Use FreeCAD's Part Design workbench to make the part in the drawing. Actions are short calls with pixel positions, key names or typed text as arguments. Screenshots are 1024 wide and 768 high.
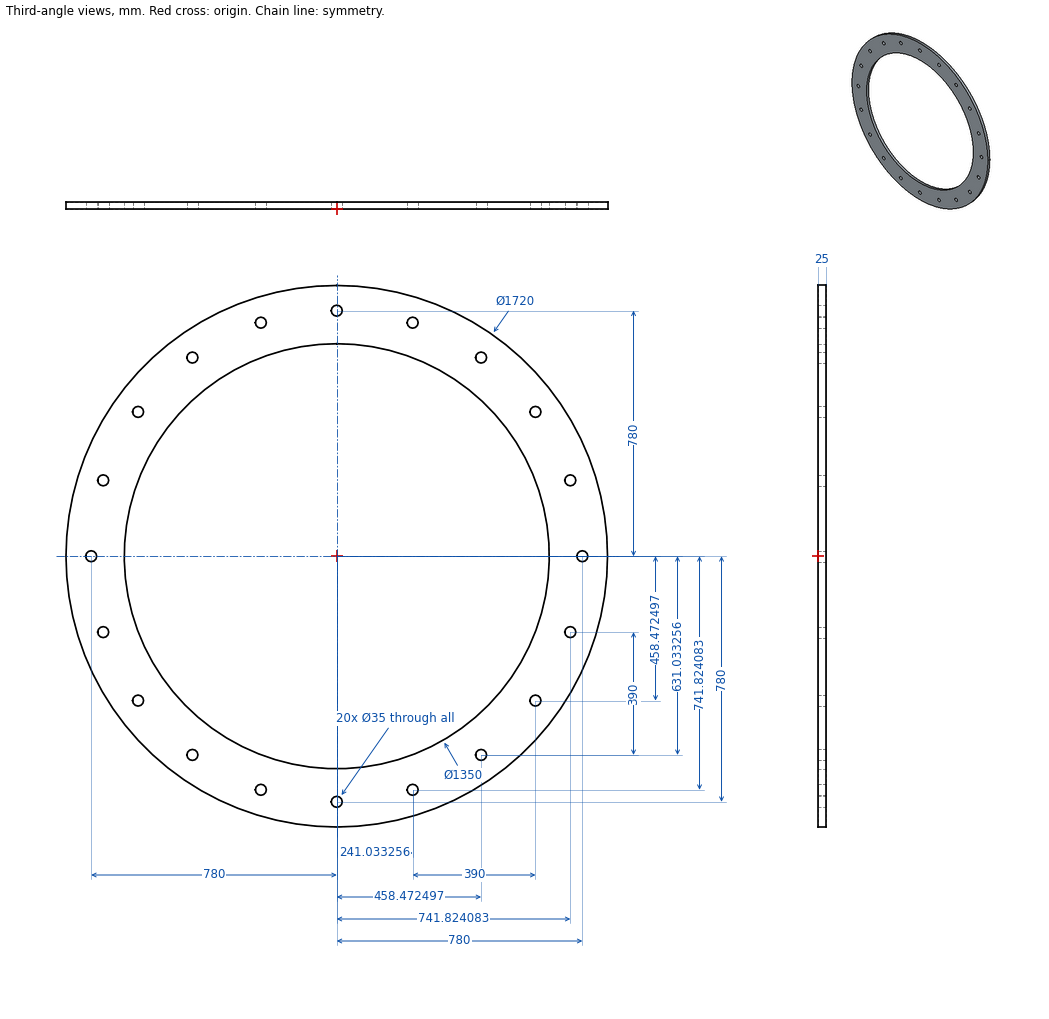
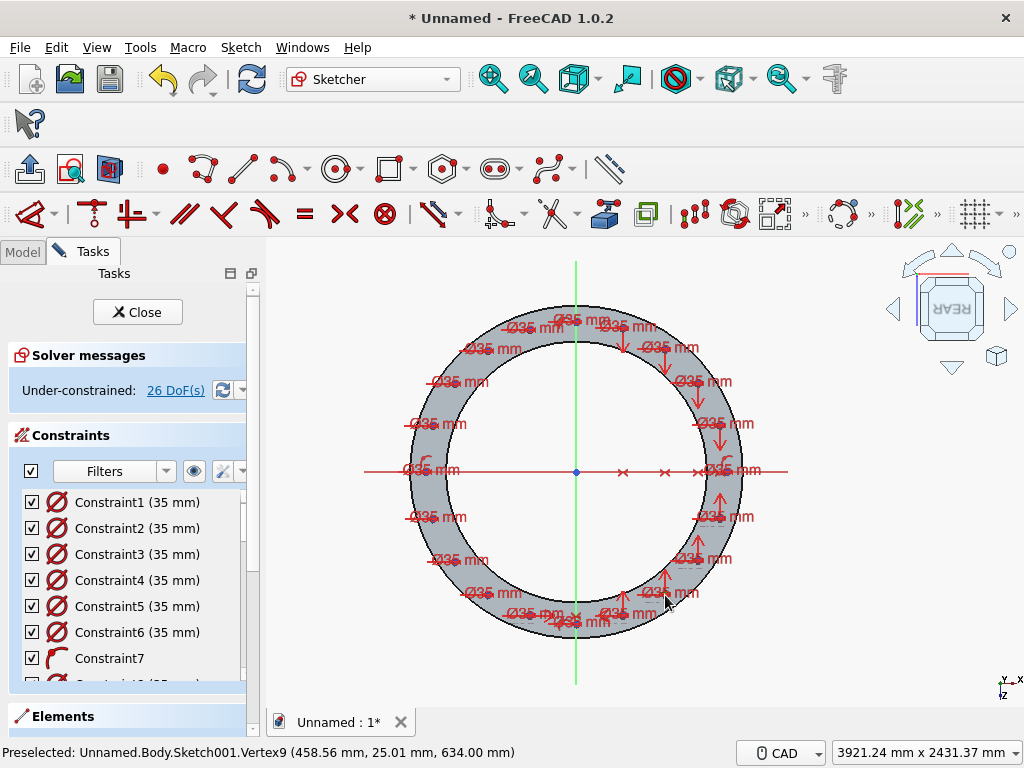
click(488, 595)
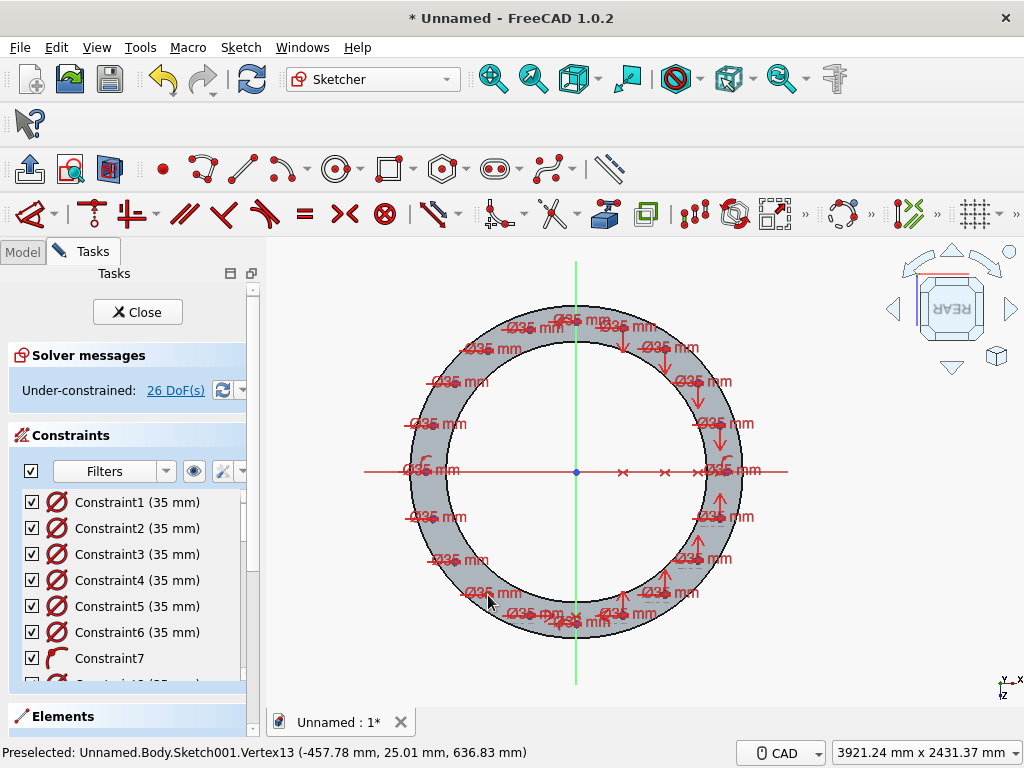
click(576, 590)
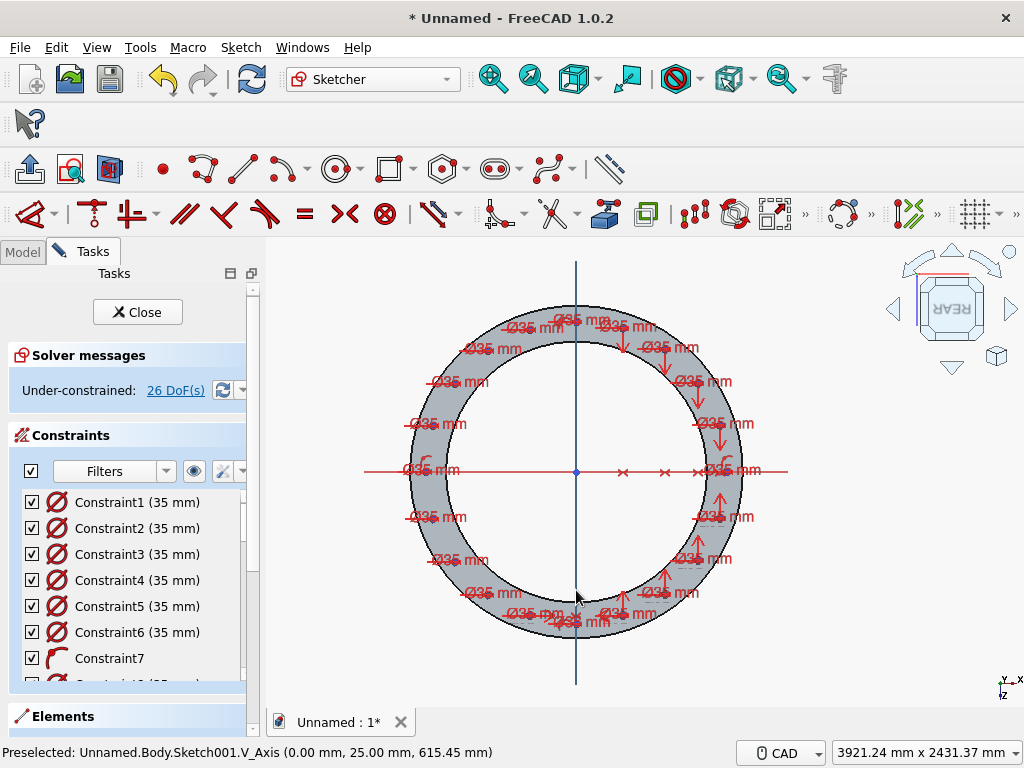
key(s)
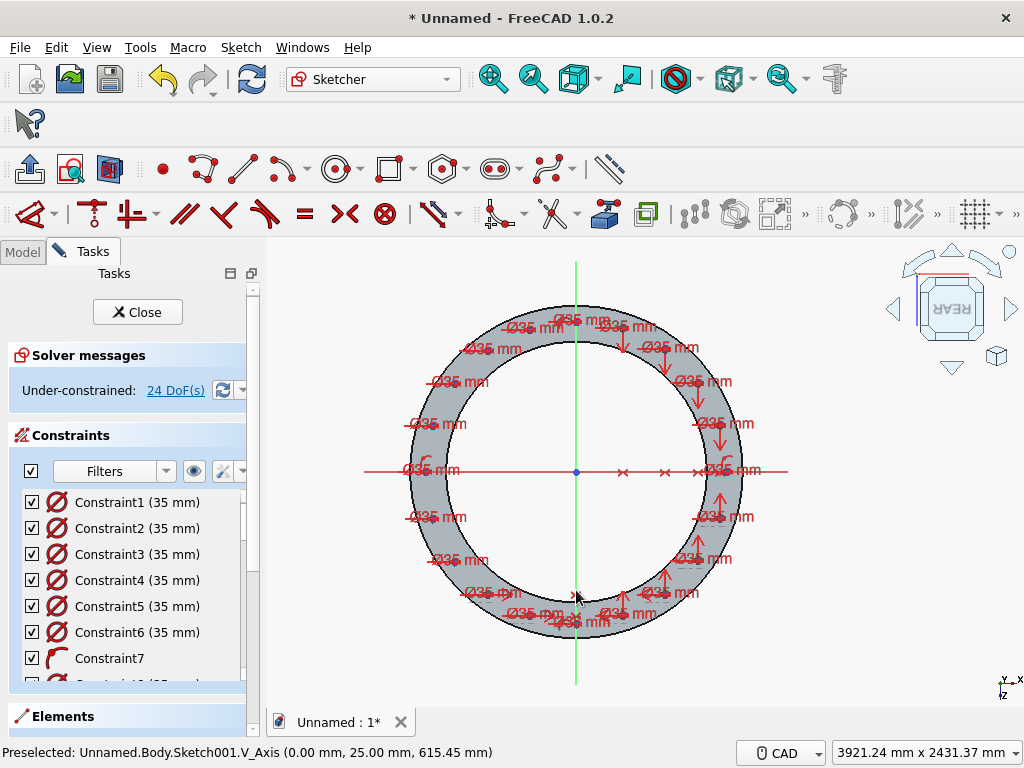
click(698, 561)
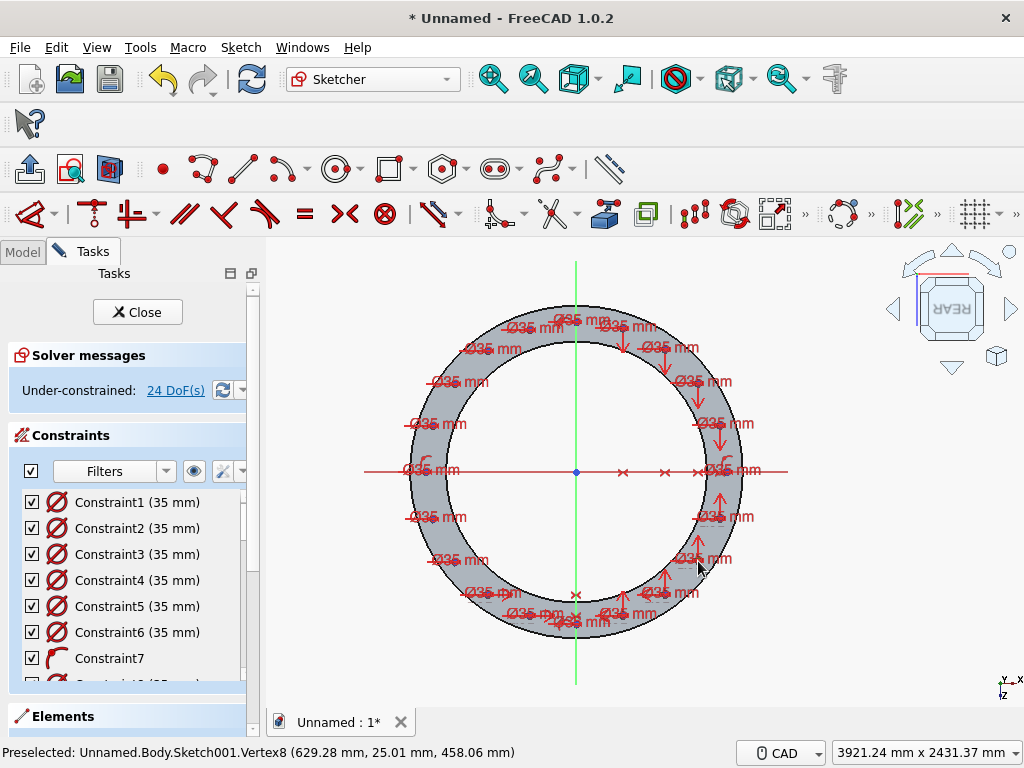
click(455, 562)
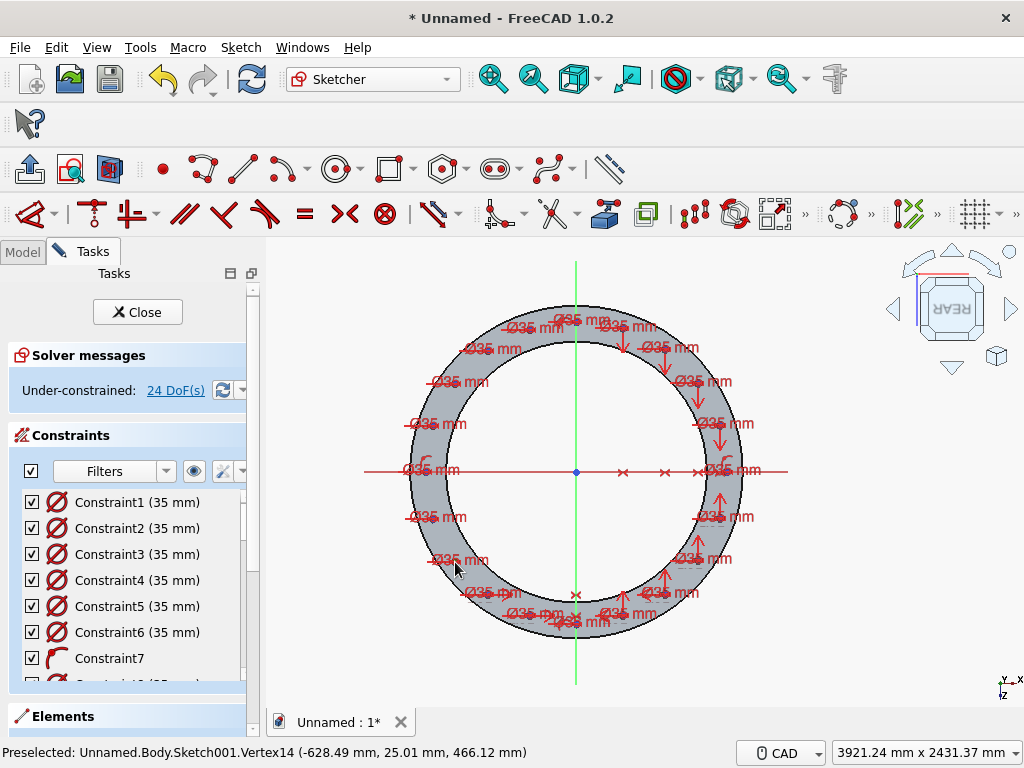
click(576, 561)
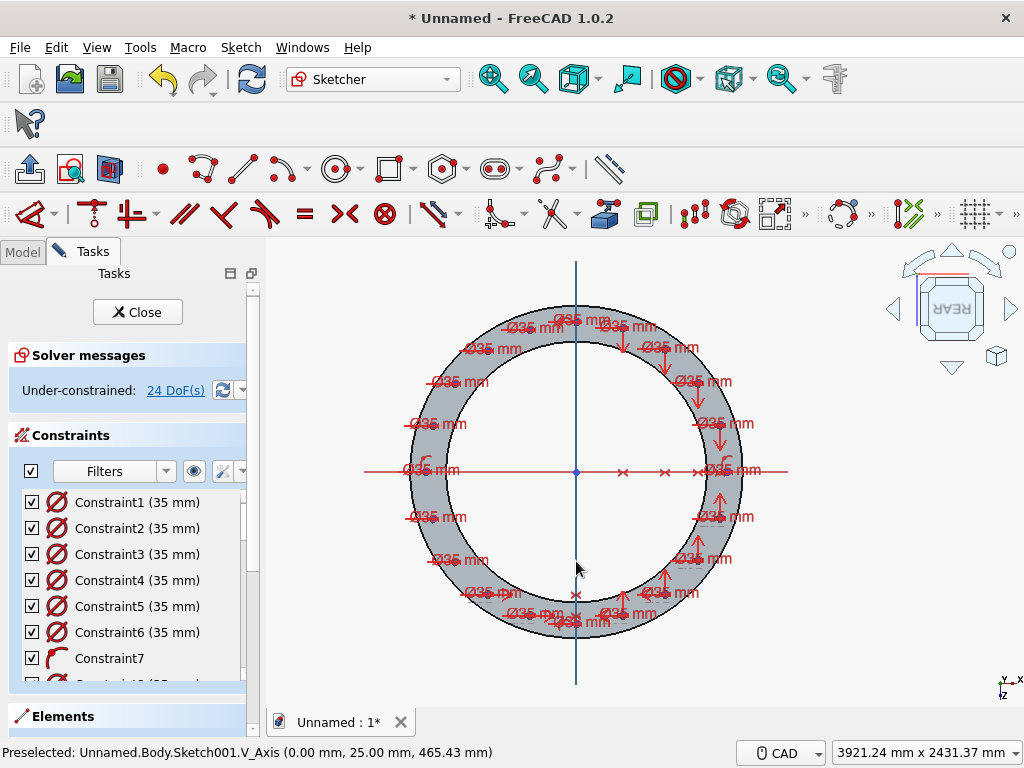
key(s)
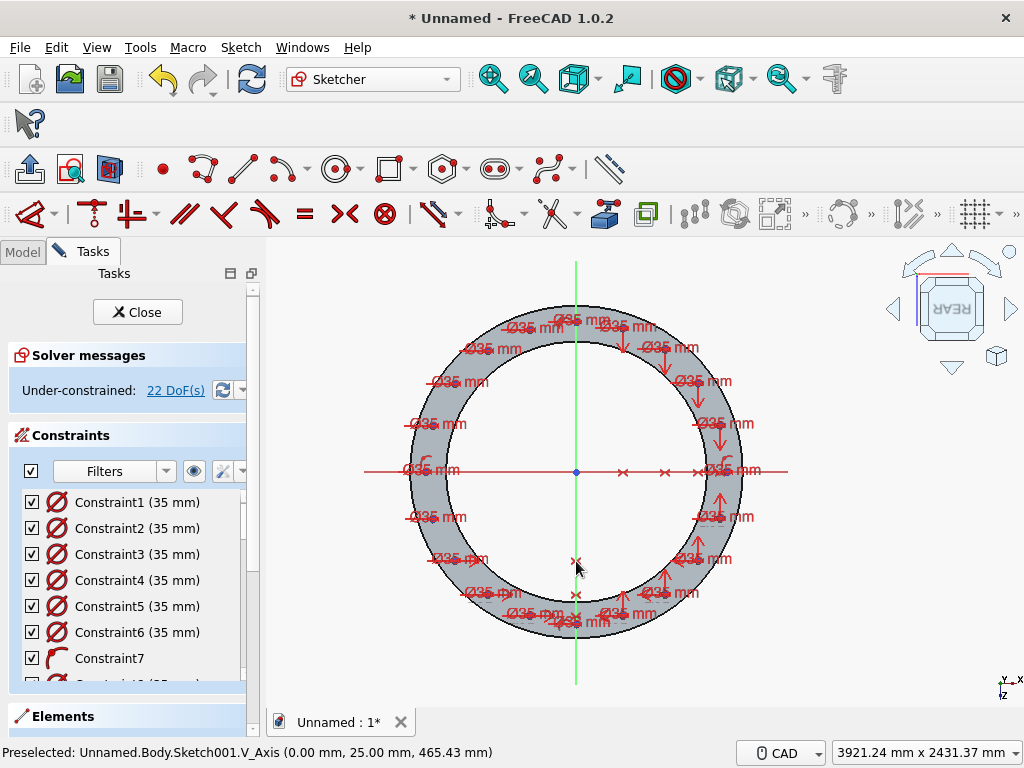
click(720, 519)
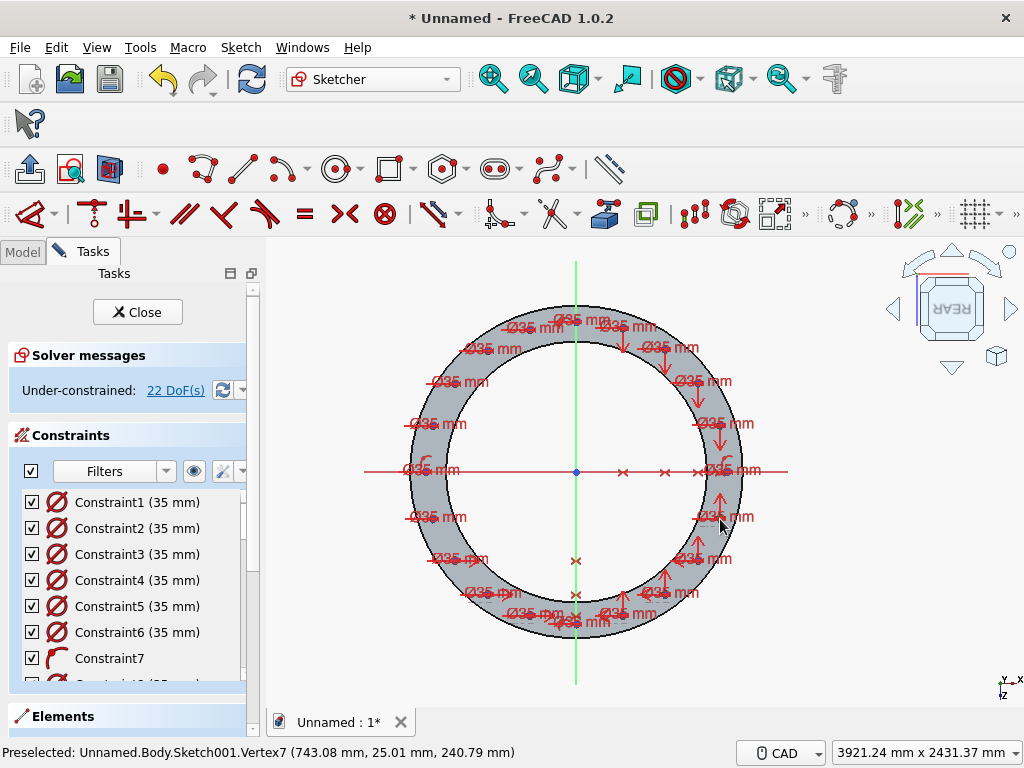
click(433, 519)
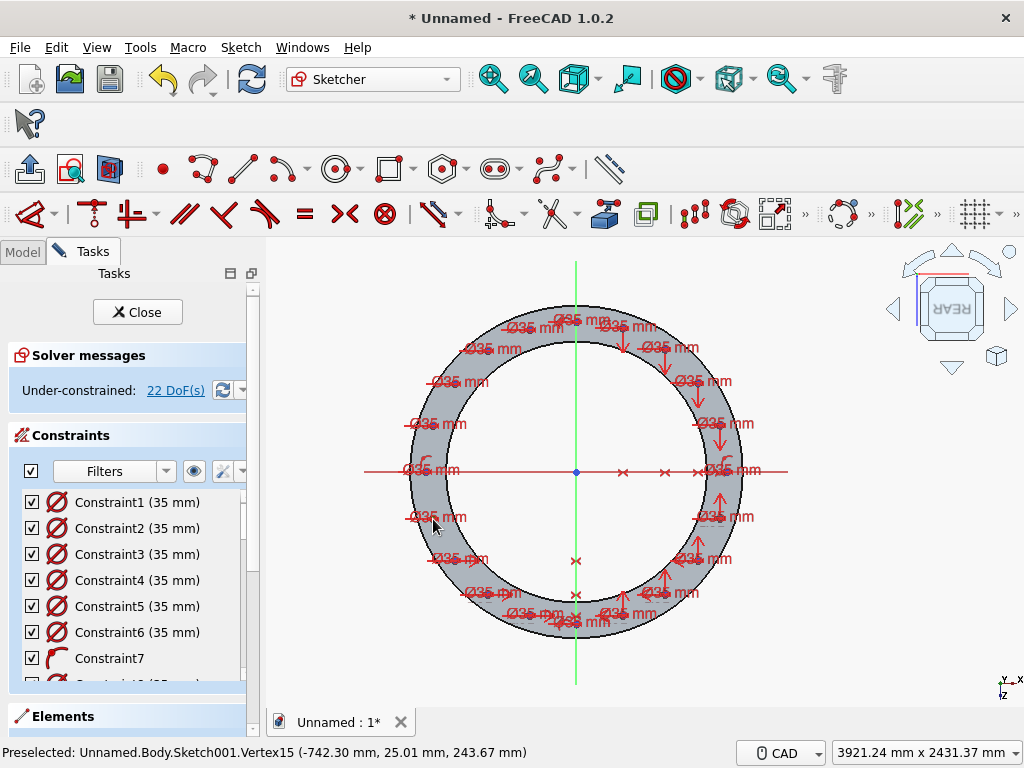
click(576, 531)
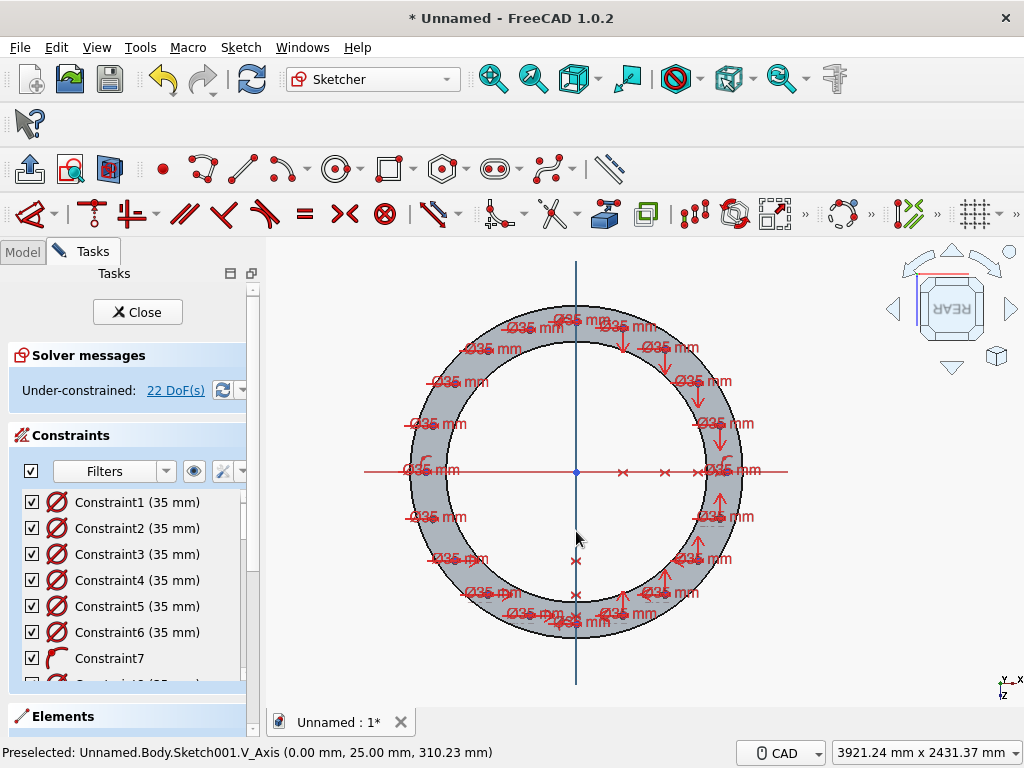
key(s)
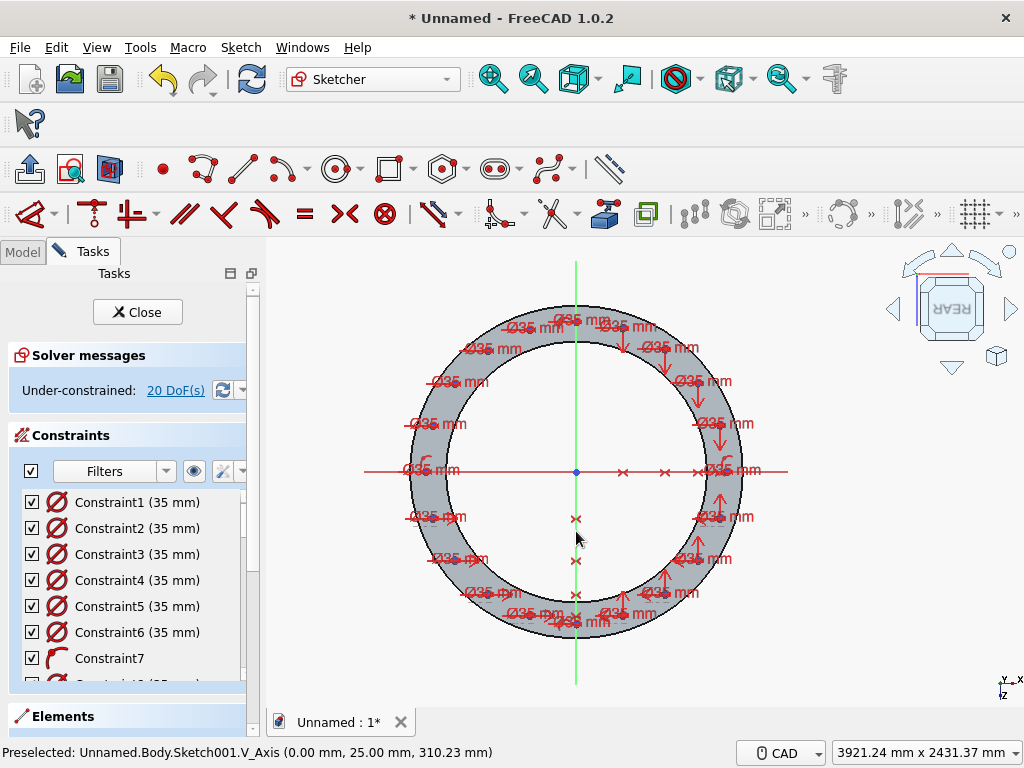
click(720, 425)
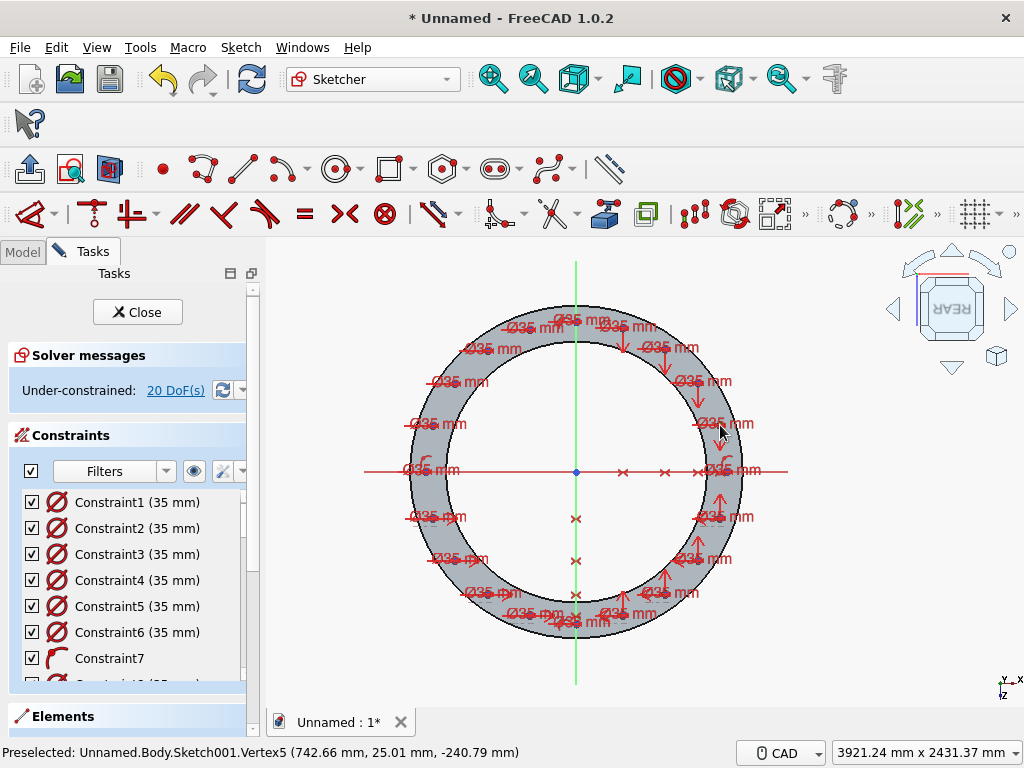
click(433, 426)